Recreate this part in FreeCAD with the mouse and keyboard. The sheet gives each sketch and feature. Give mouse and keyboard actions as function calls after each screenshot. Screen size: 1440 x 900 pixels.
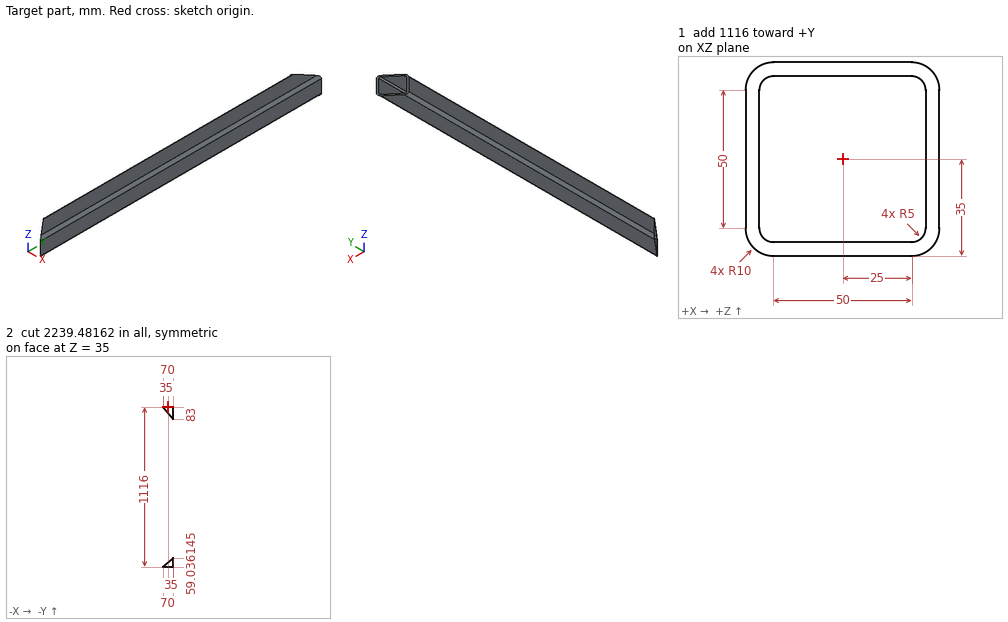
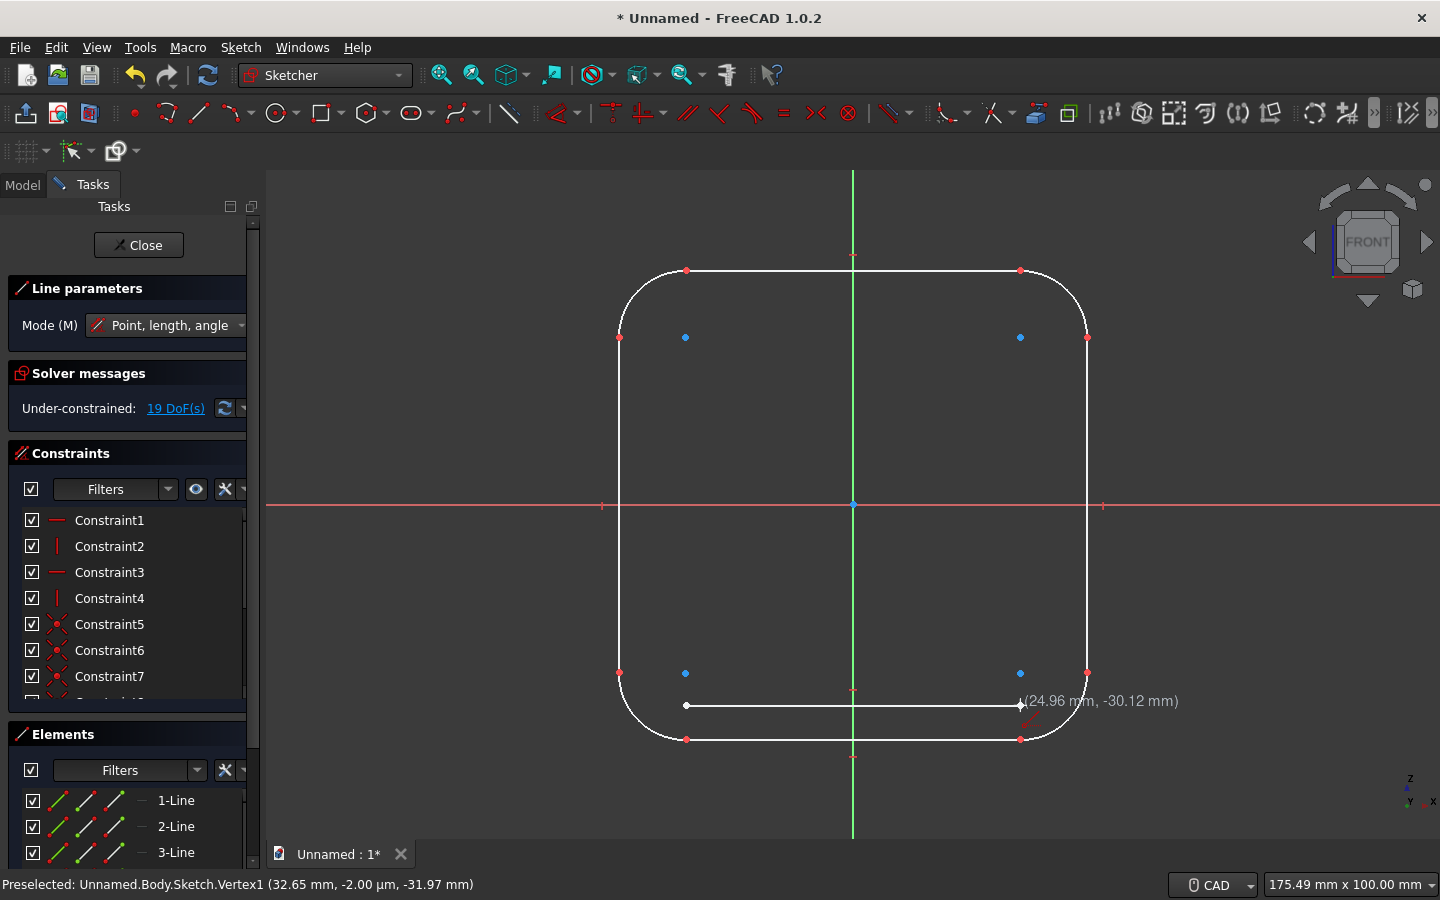
click(1054, 672)
click(1054, 337)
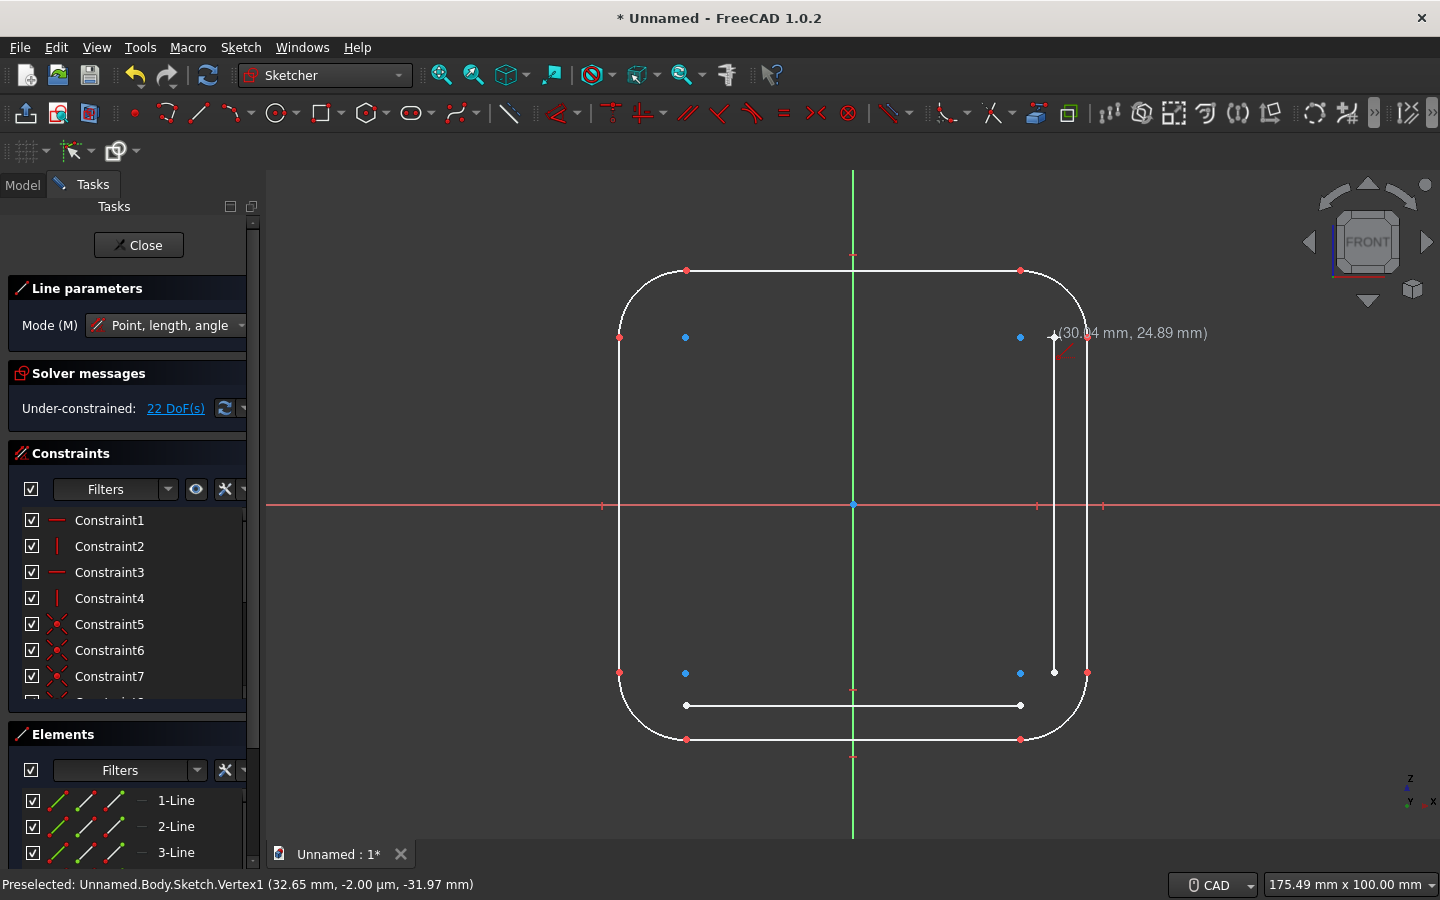
click(1020, 304)
click(686, 304)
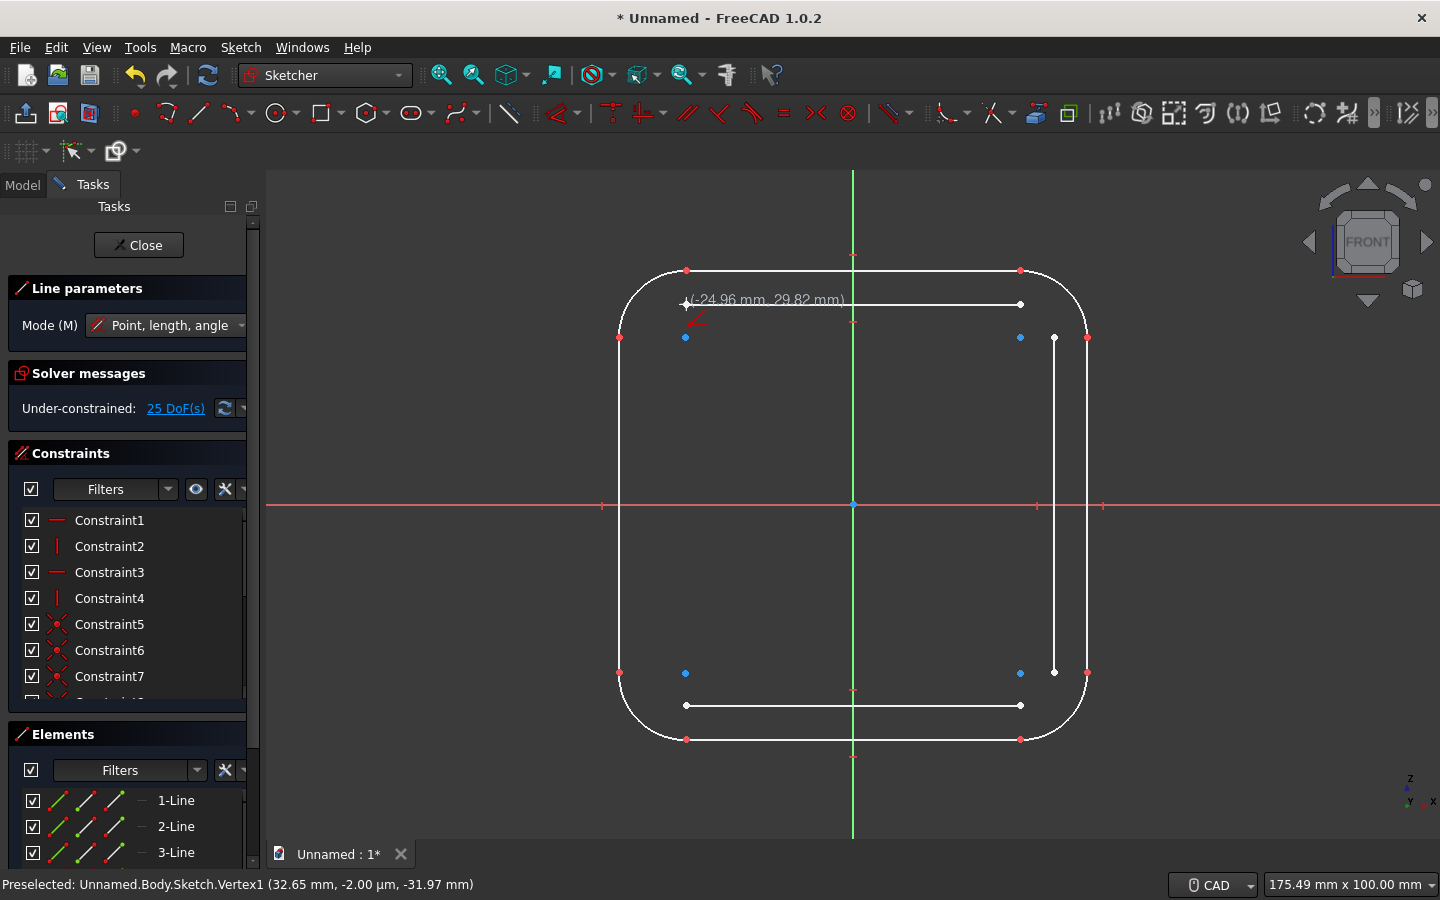
click(652, 337)
click(652, 672)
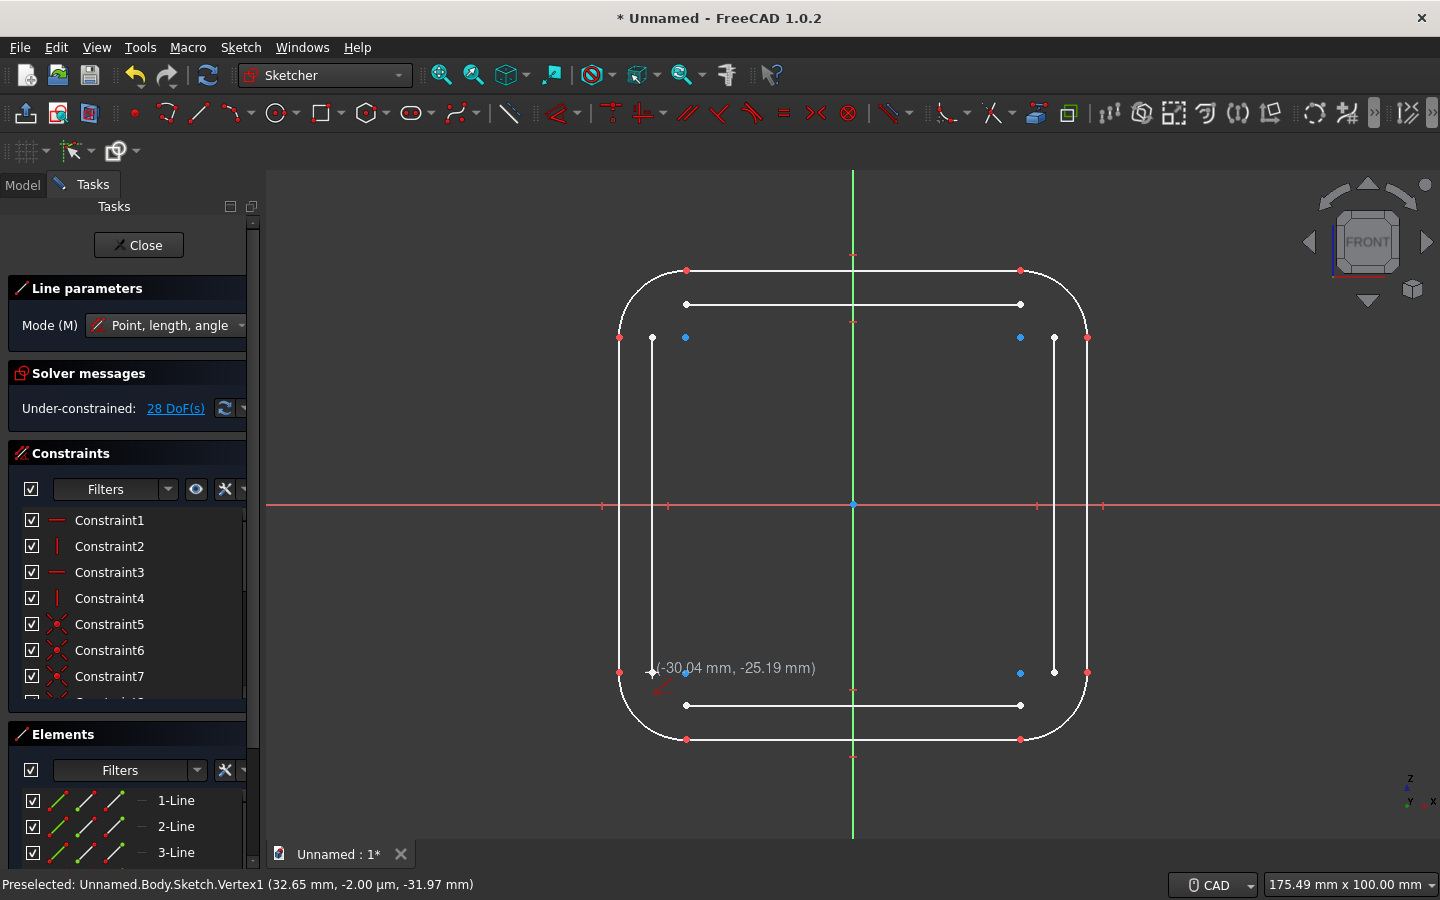
key(g)
key(3)
key(a)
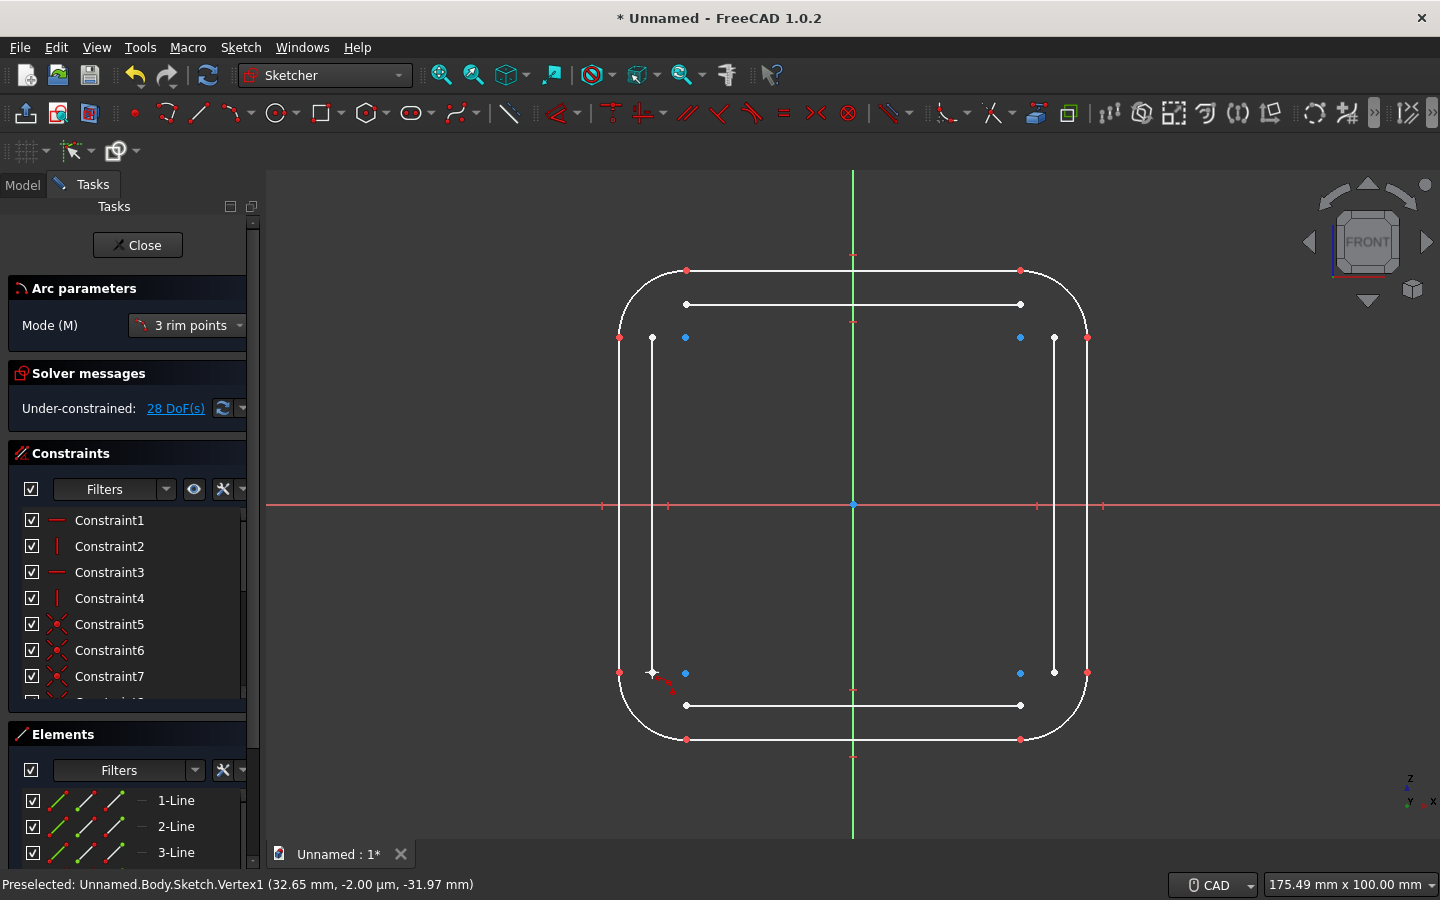
click(1020, 706)
click(1054, 673)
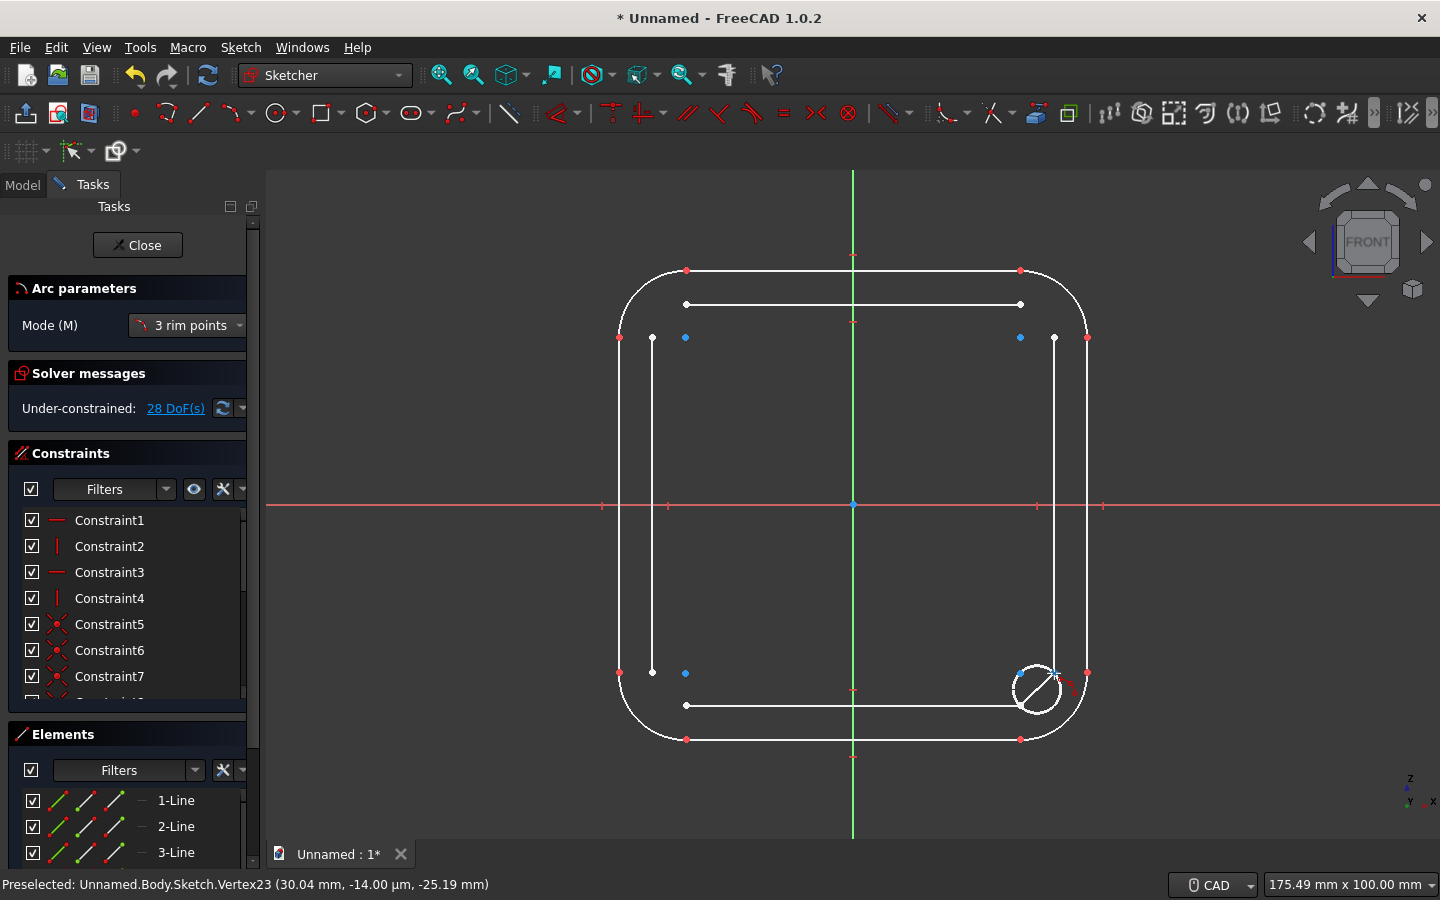
scroll(1044, 695, up, 3)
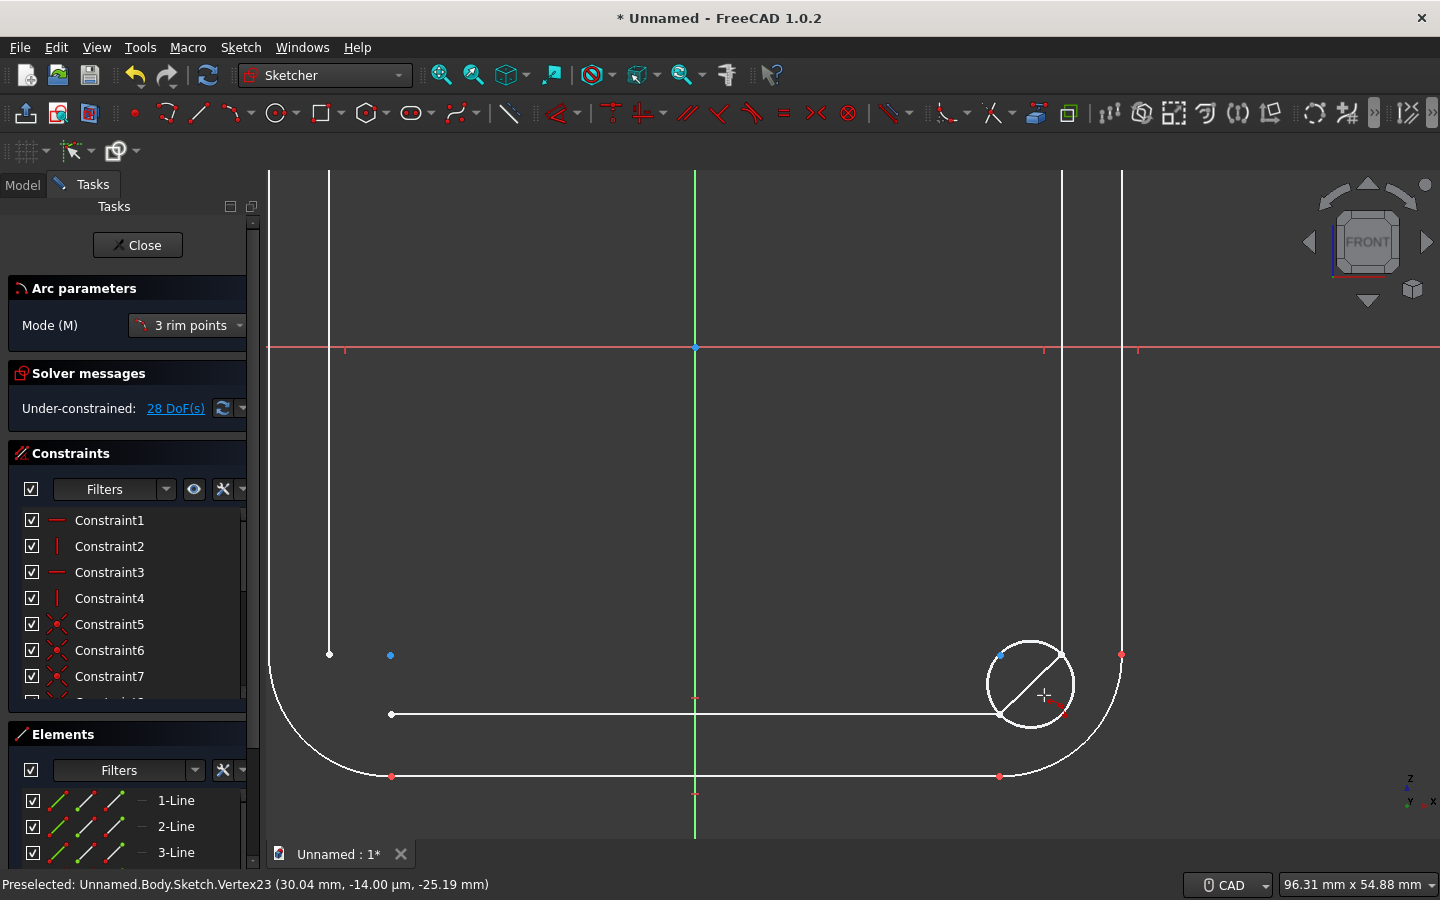
click(1043, 695)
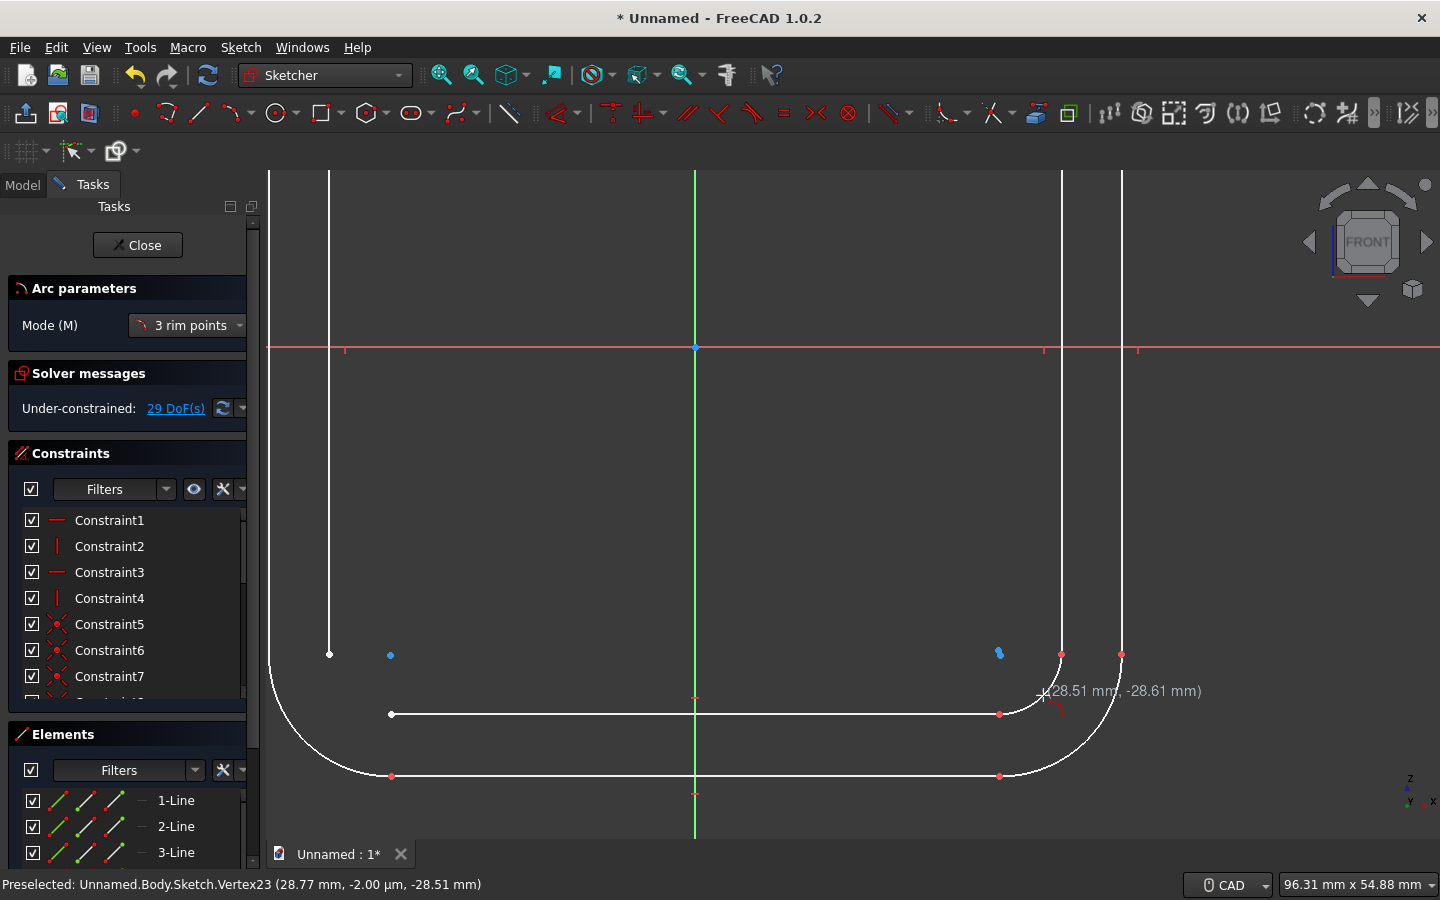
scroll(893, 696, down, 3)